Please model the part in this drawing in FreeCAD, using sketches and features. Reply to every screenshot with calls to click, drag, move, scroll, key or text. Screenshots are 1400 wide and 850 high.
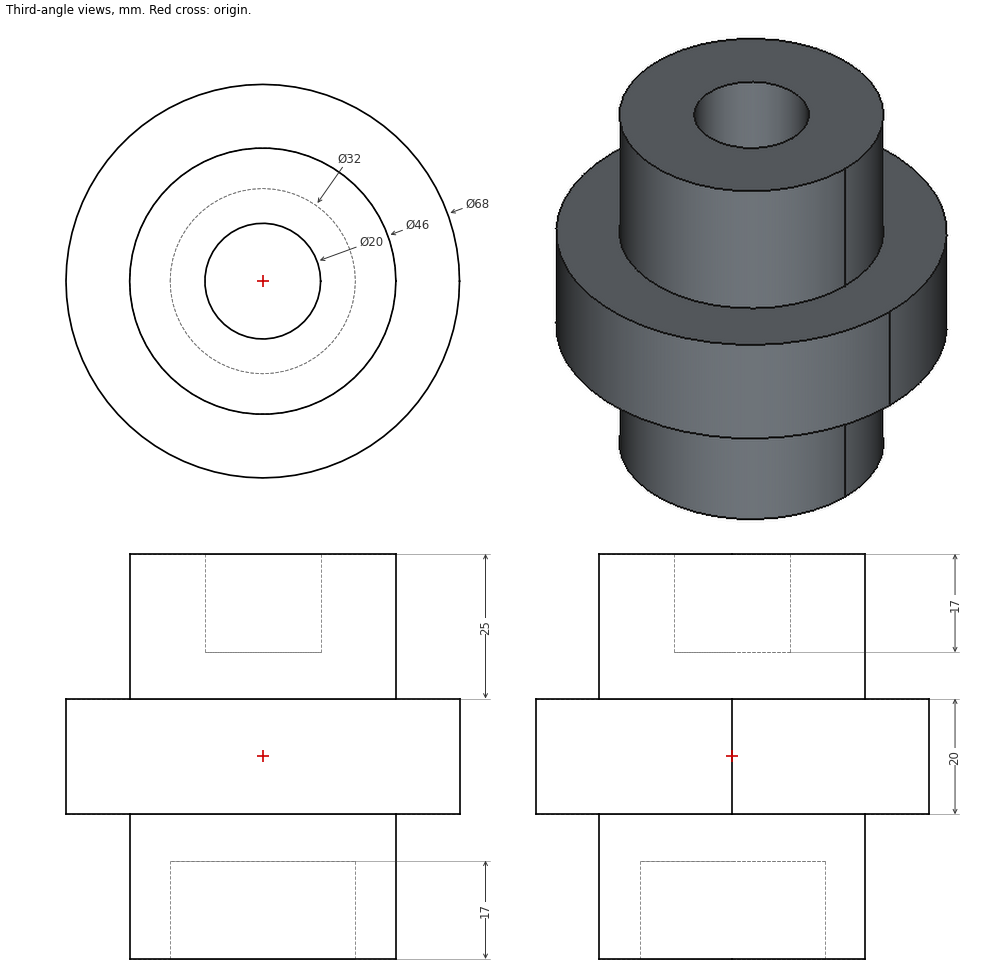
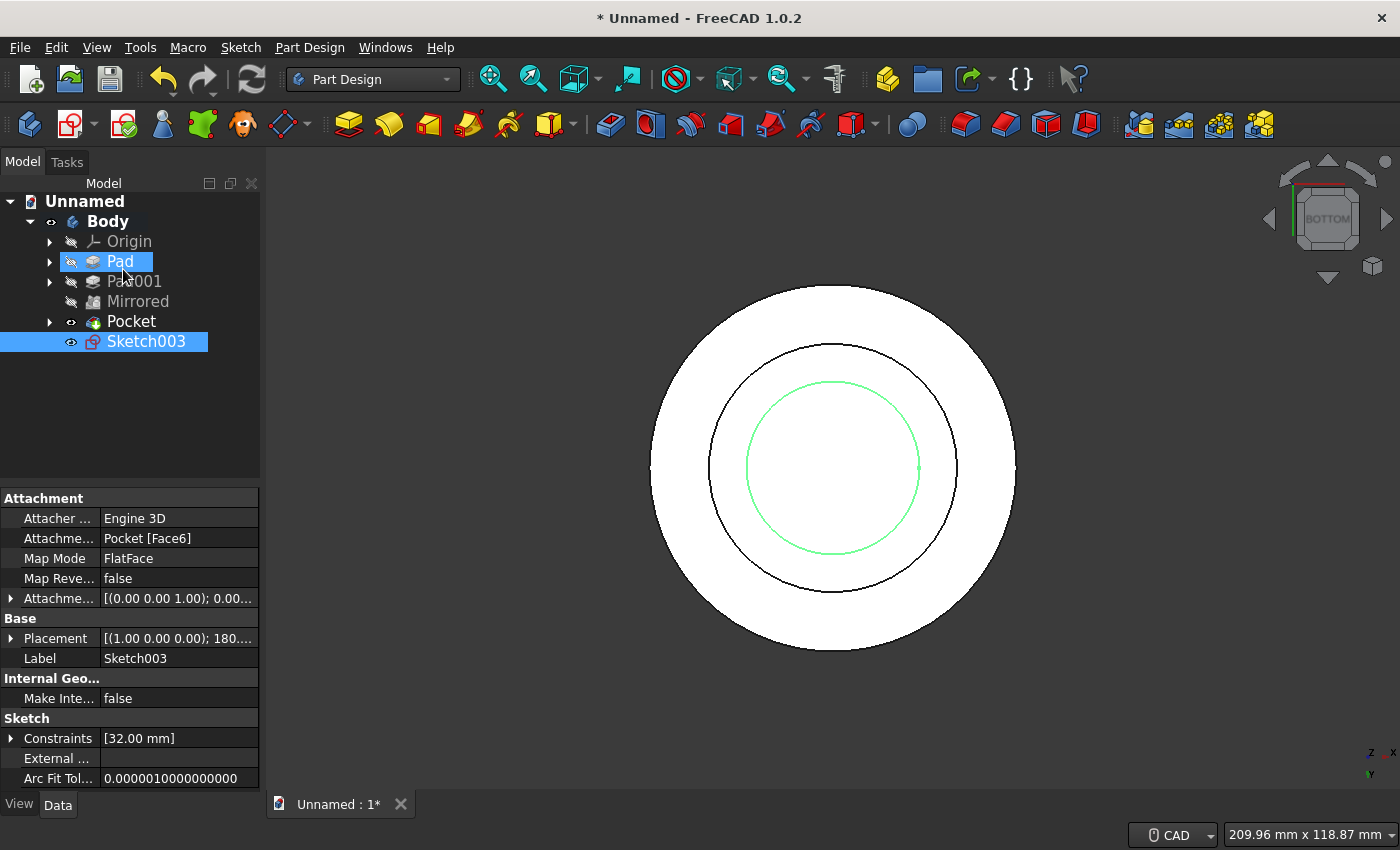
click(612, 124)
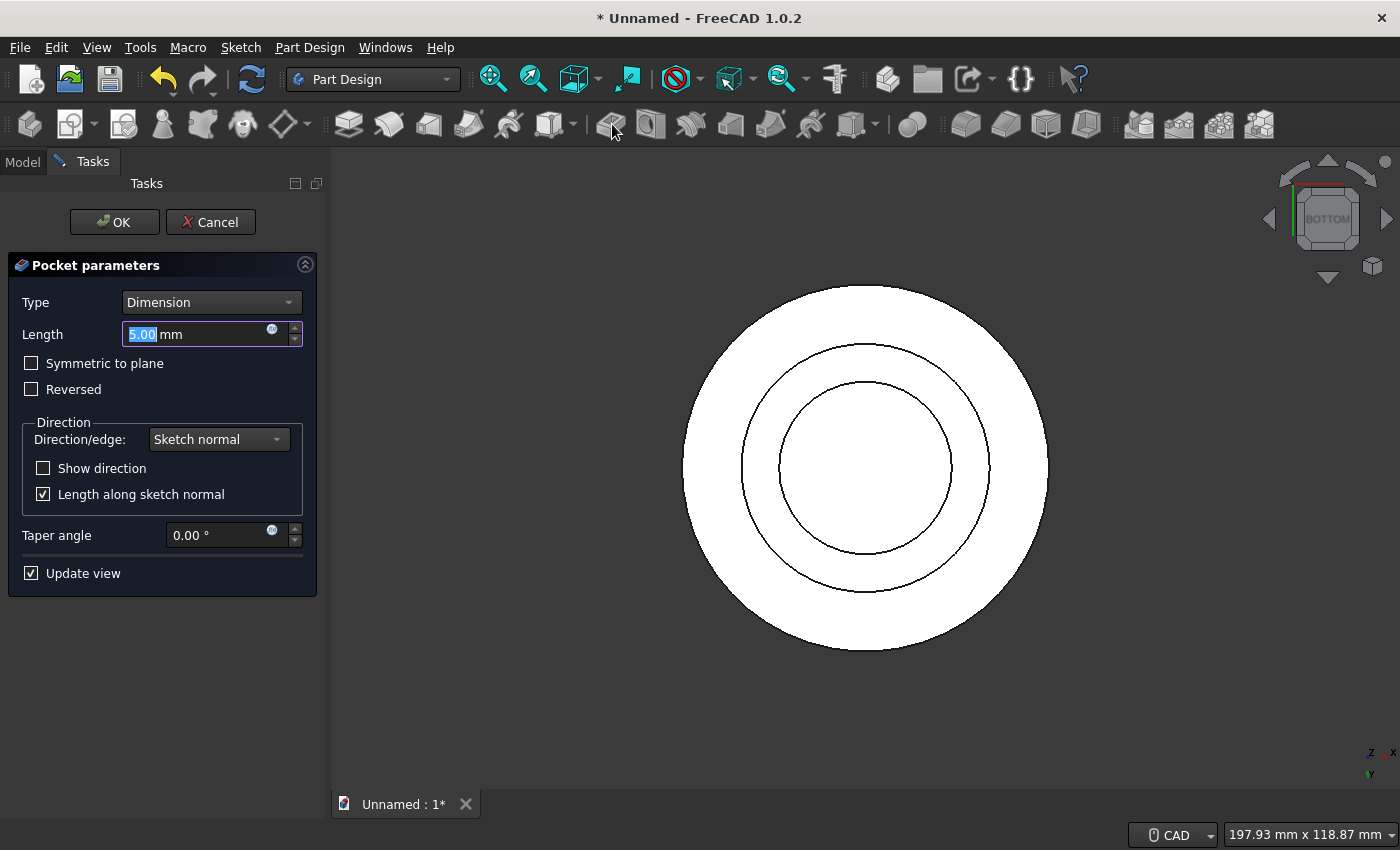
text(17)
key(Tab)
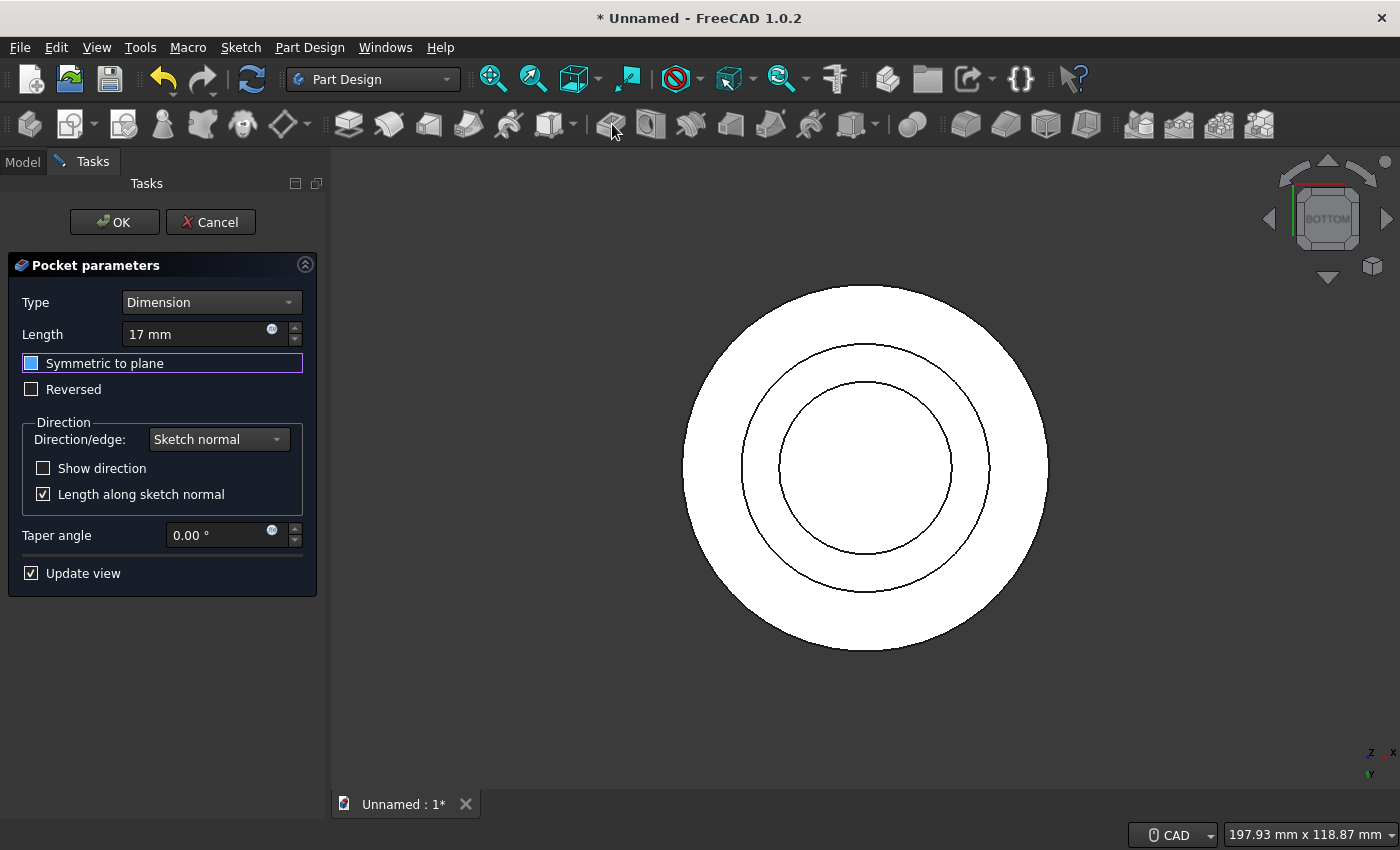
click(115, 222)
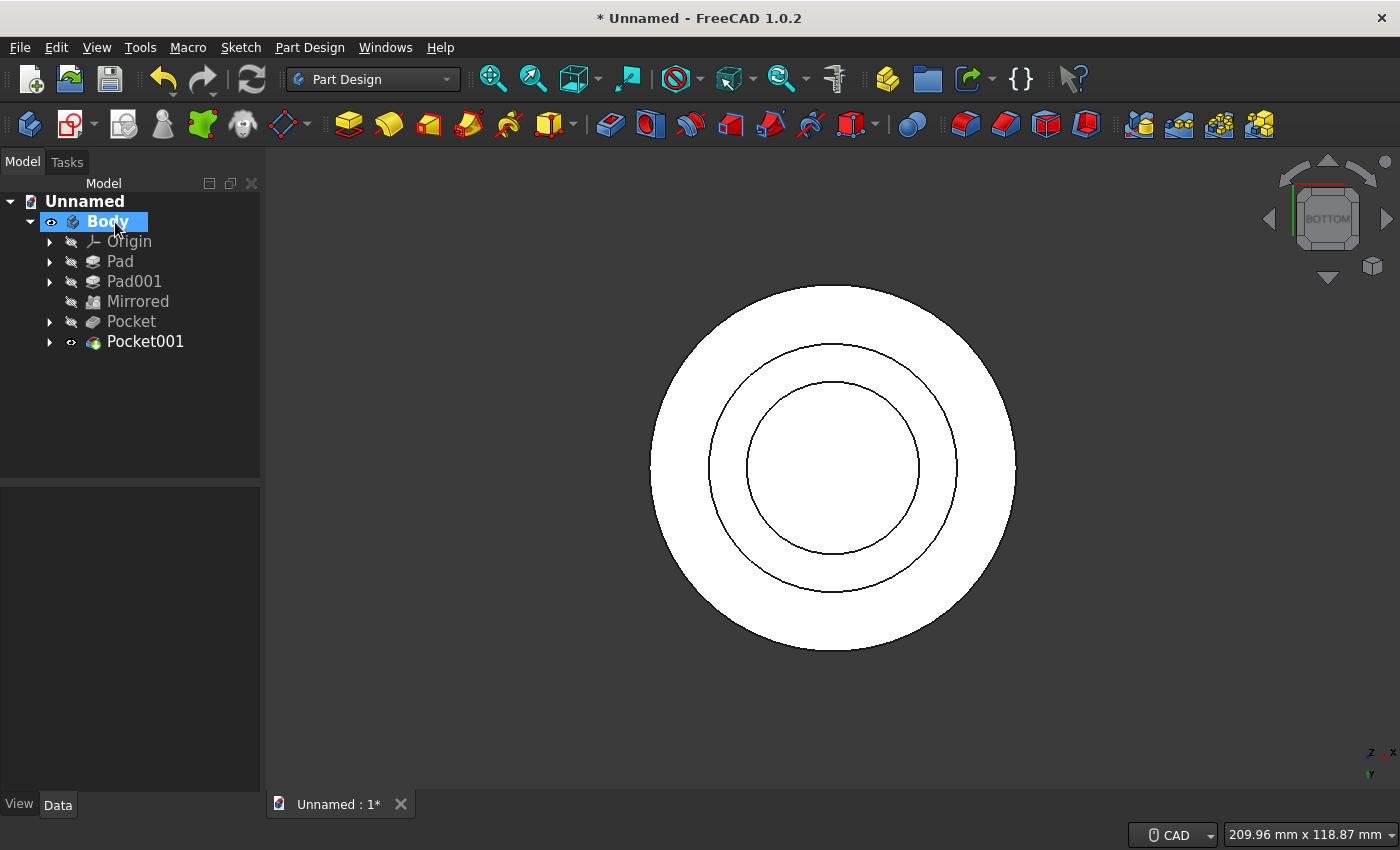
key(0)